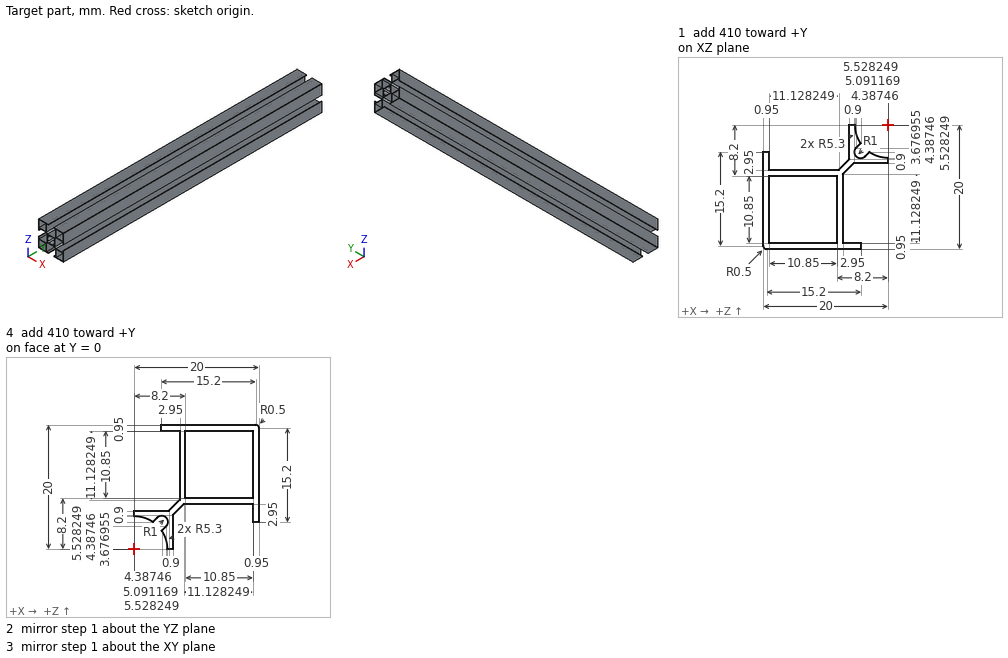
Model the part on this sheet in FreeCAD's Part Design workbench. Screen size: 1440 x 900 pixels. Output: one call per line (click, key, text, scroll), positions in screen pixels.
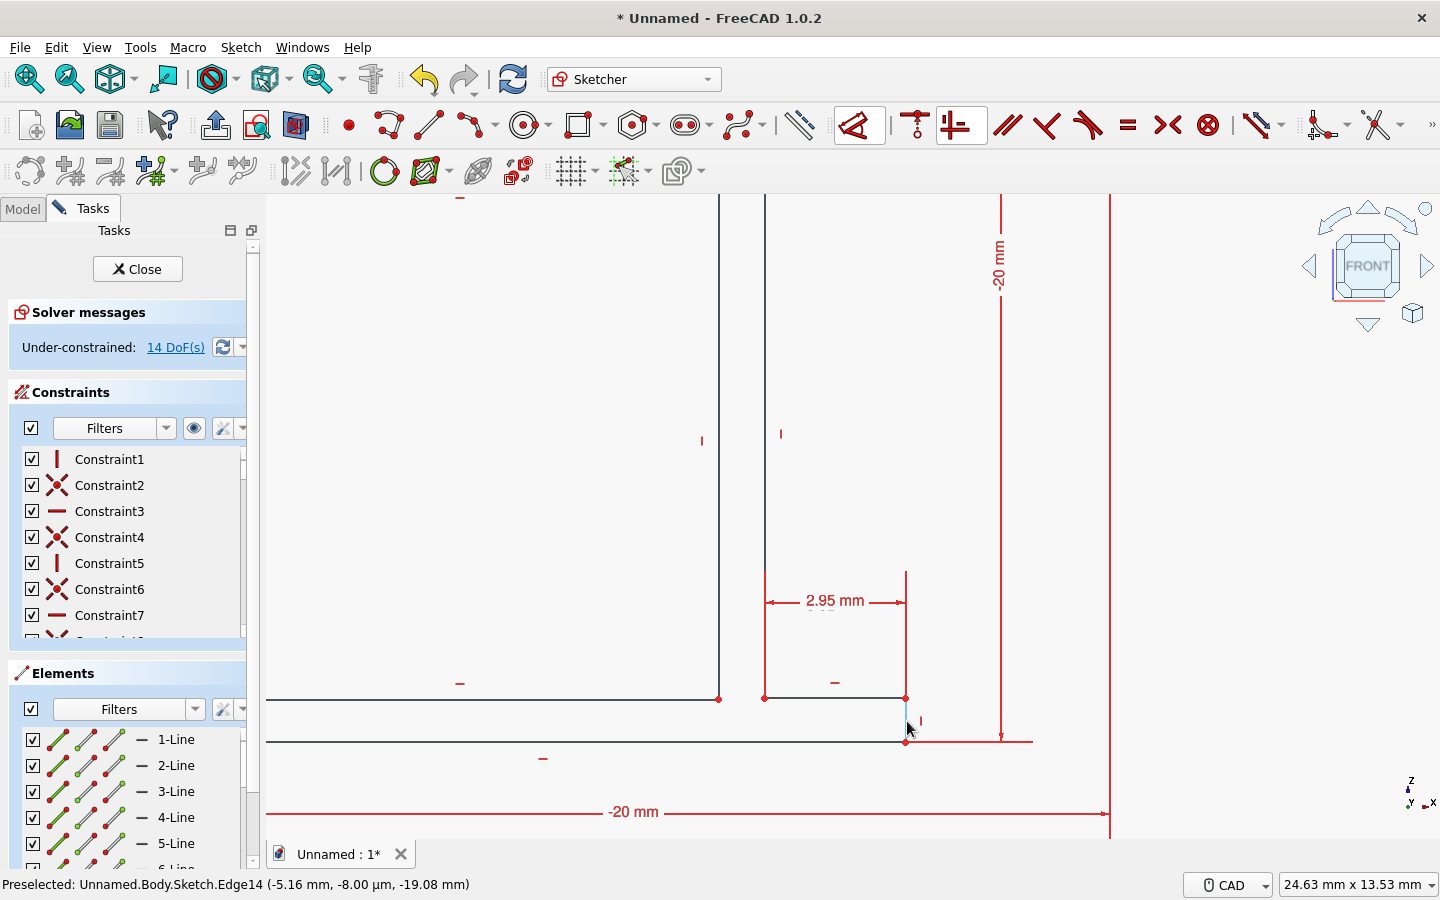
click(906, 720)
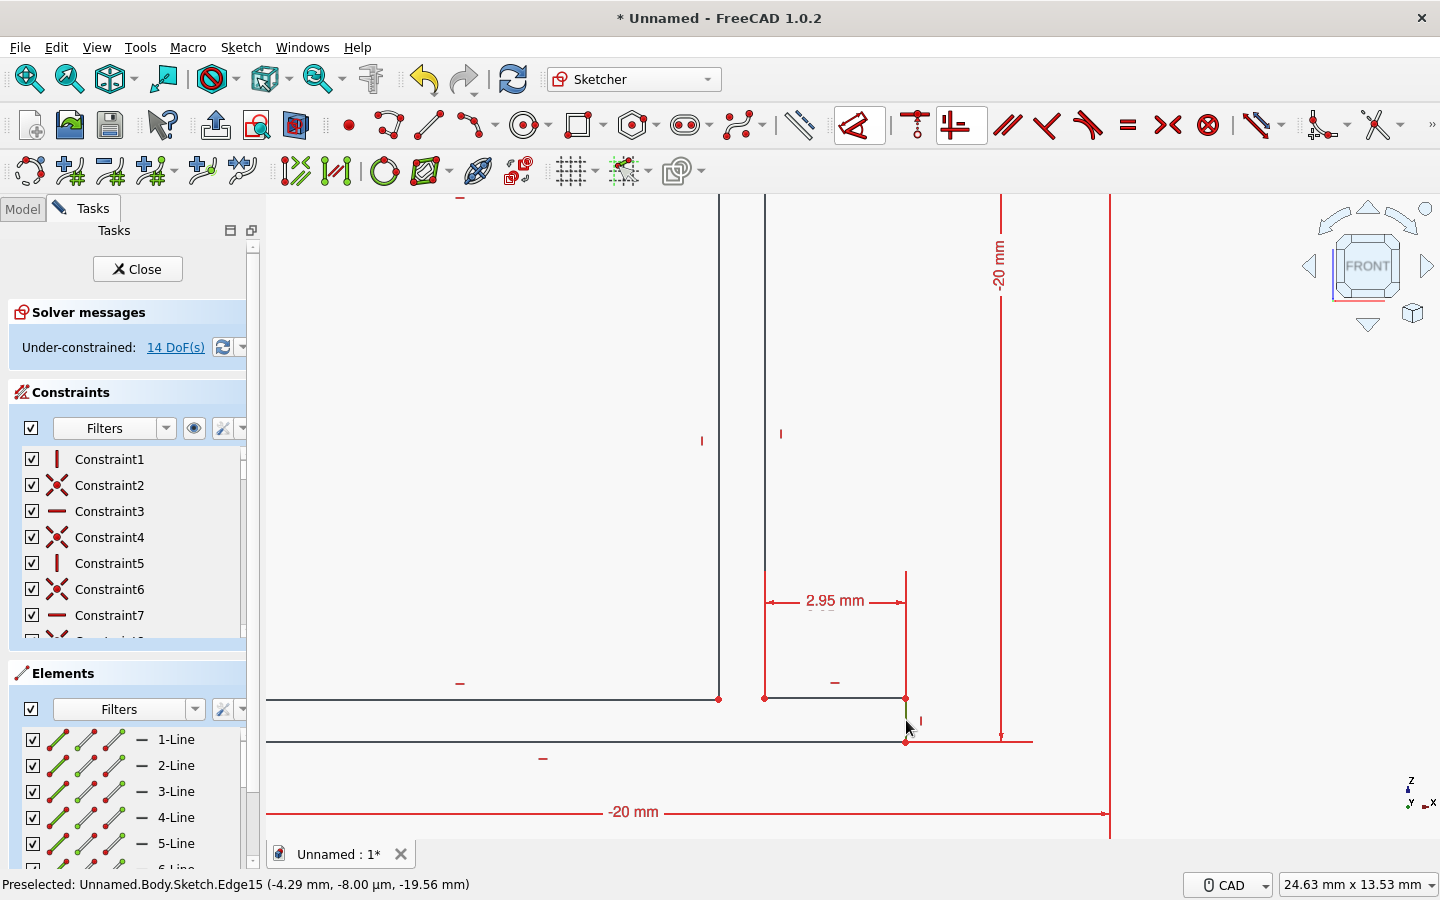
click(880, 126)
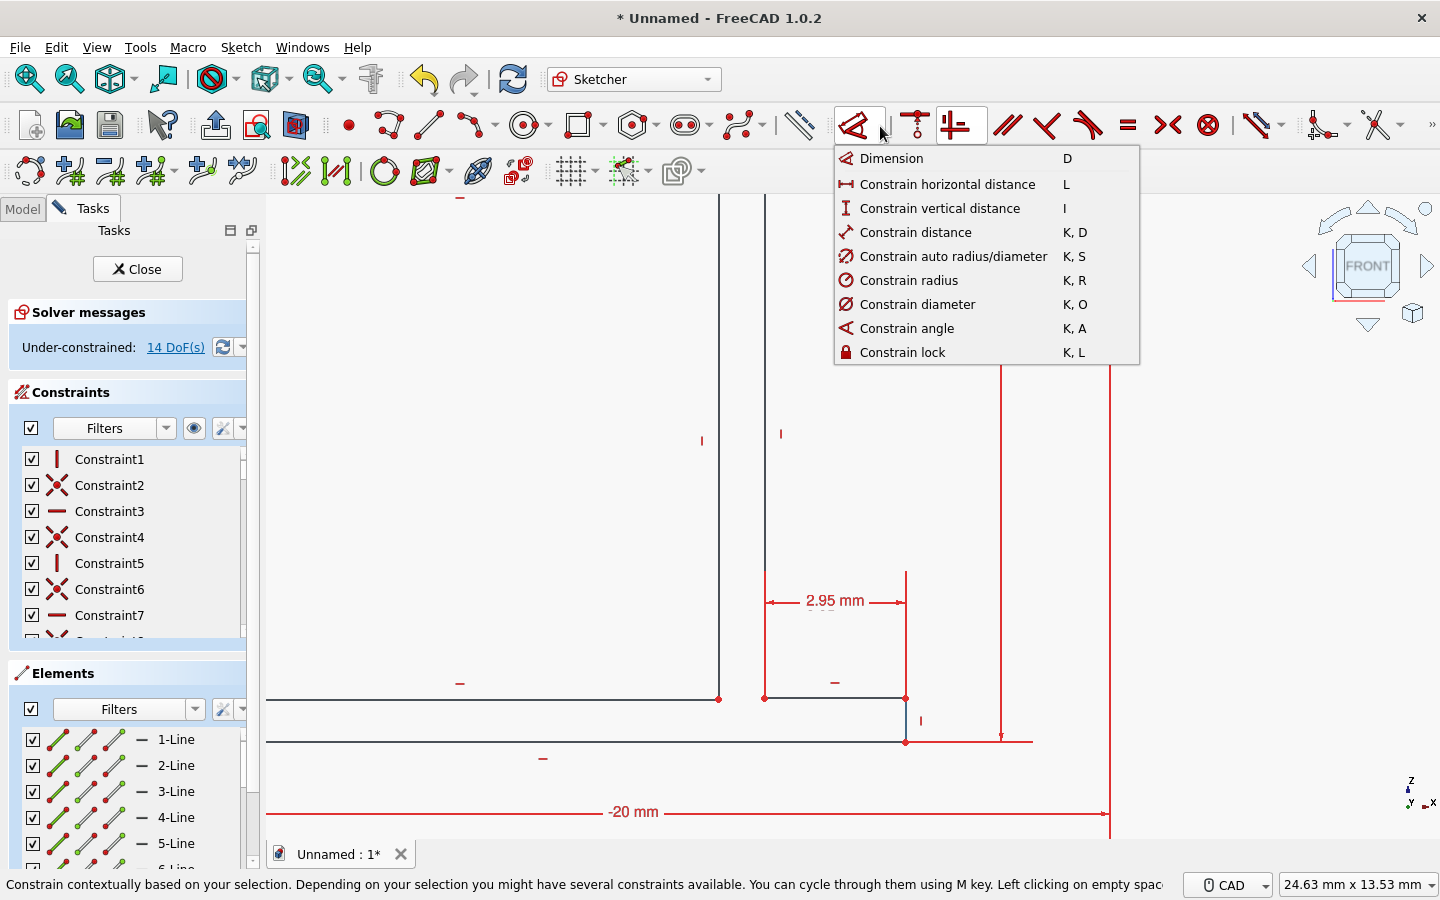
click(987, 208)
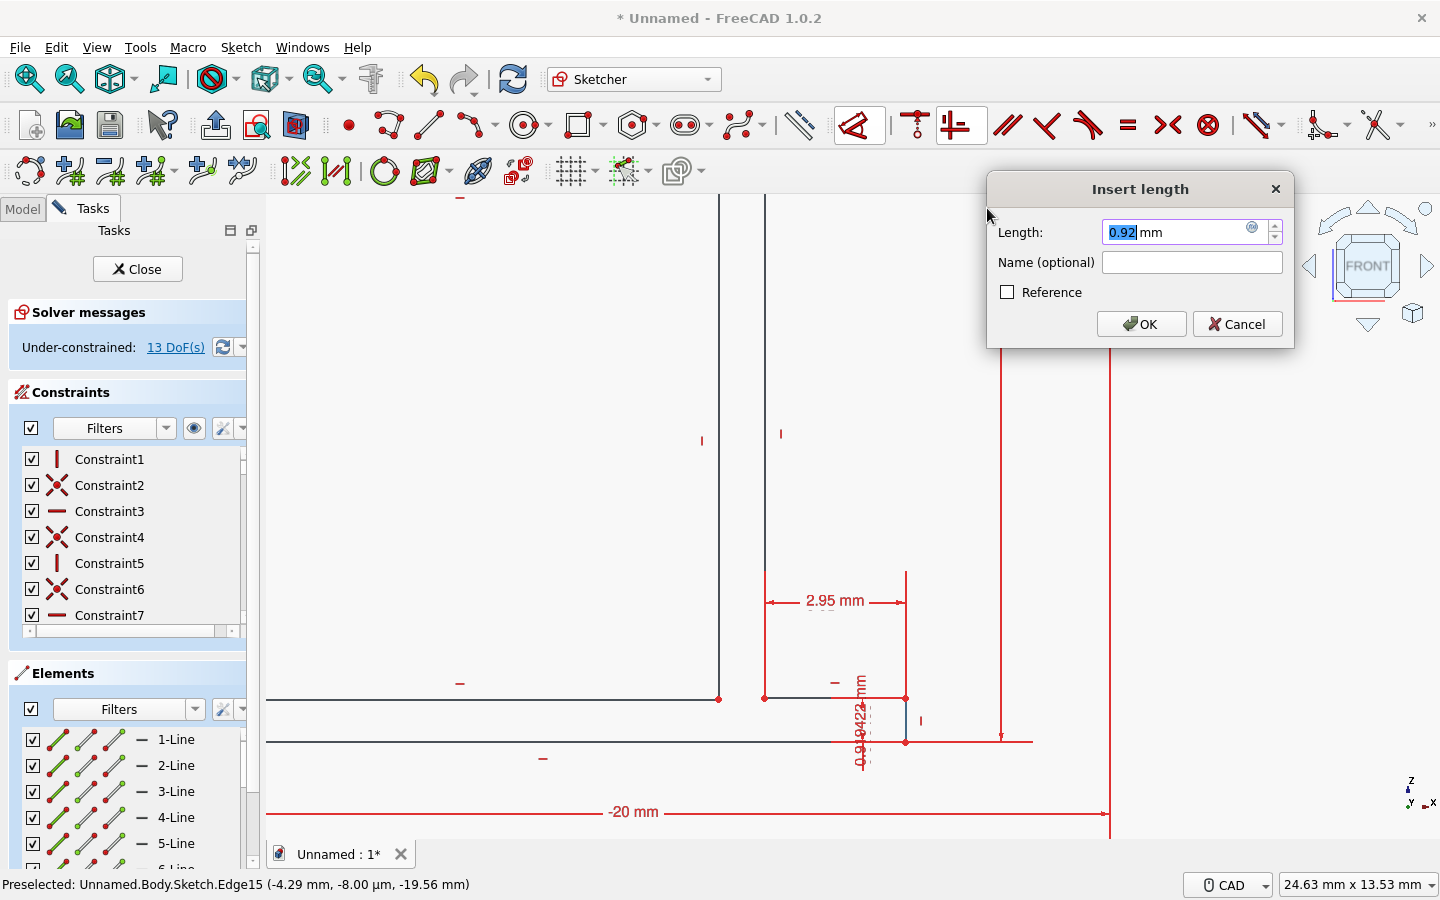
text(0.95)
key(Return)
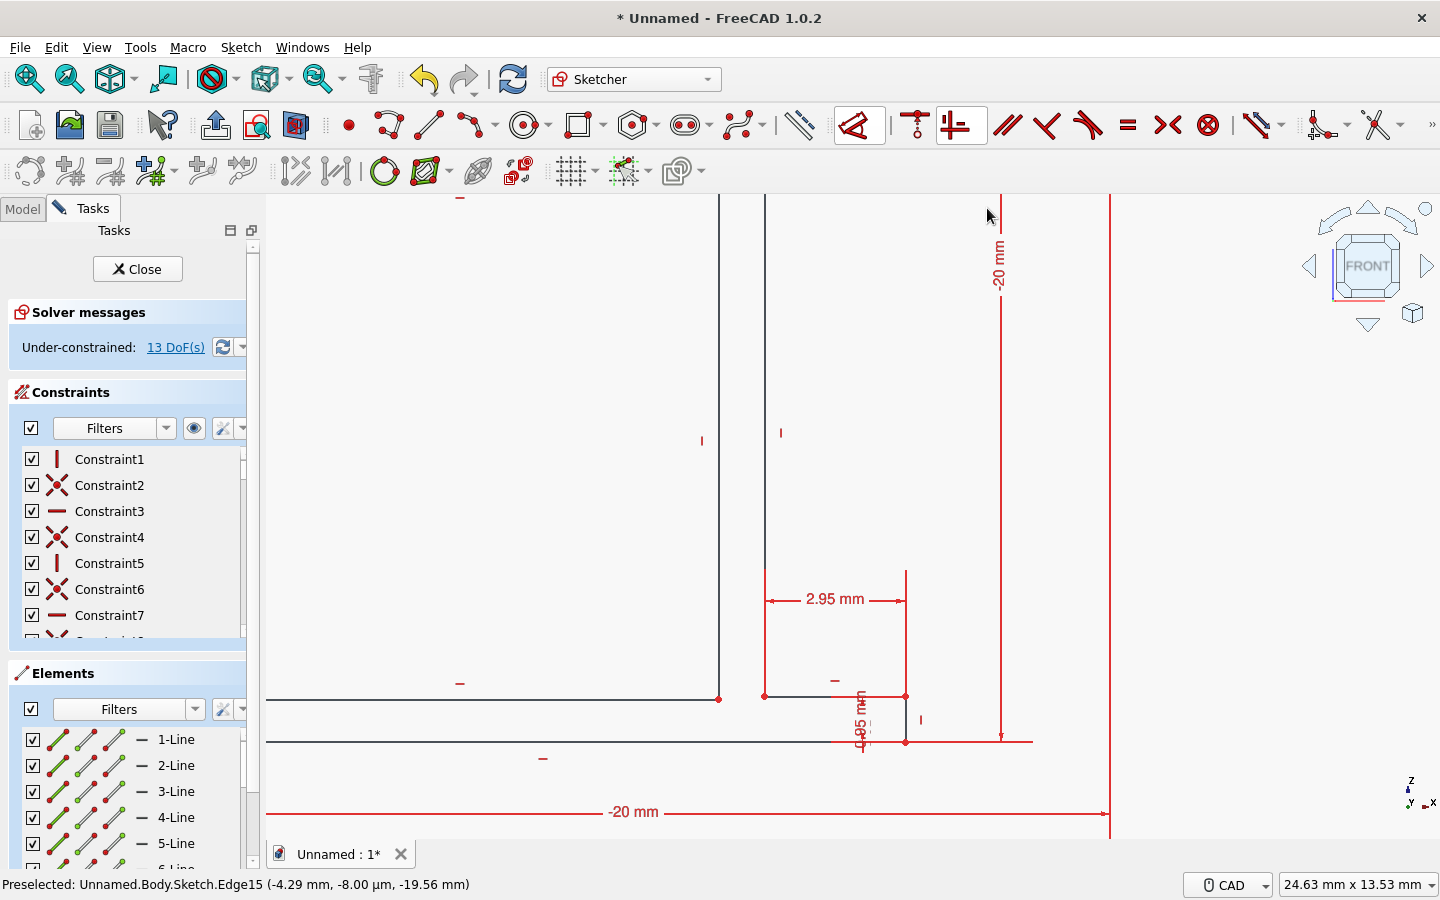
click(688, 742)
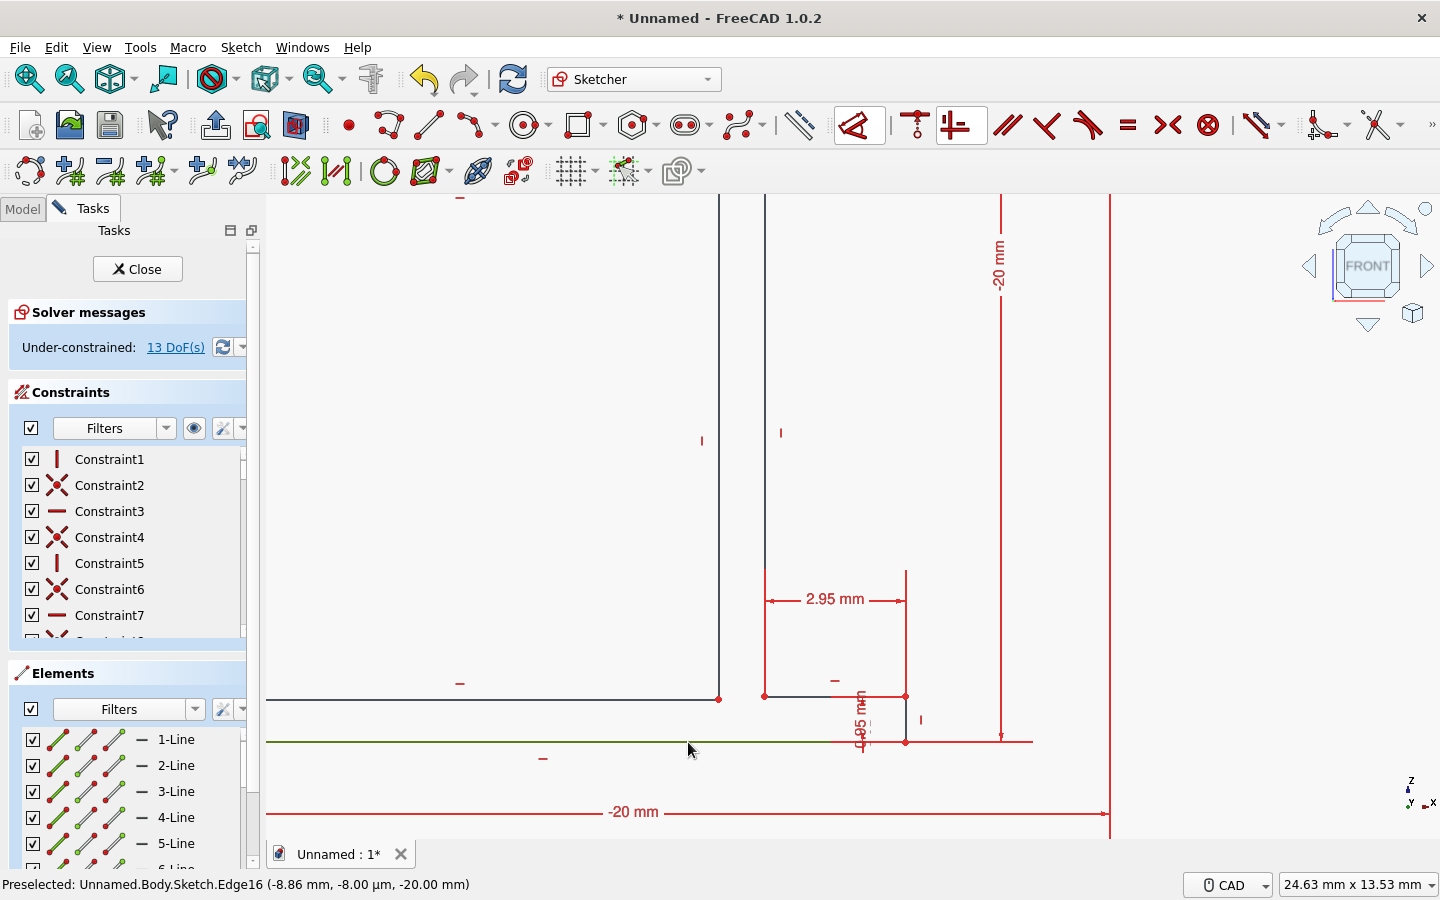
click(880, 126)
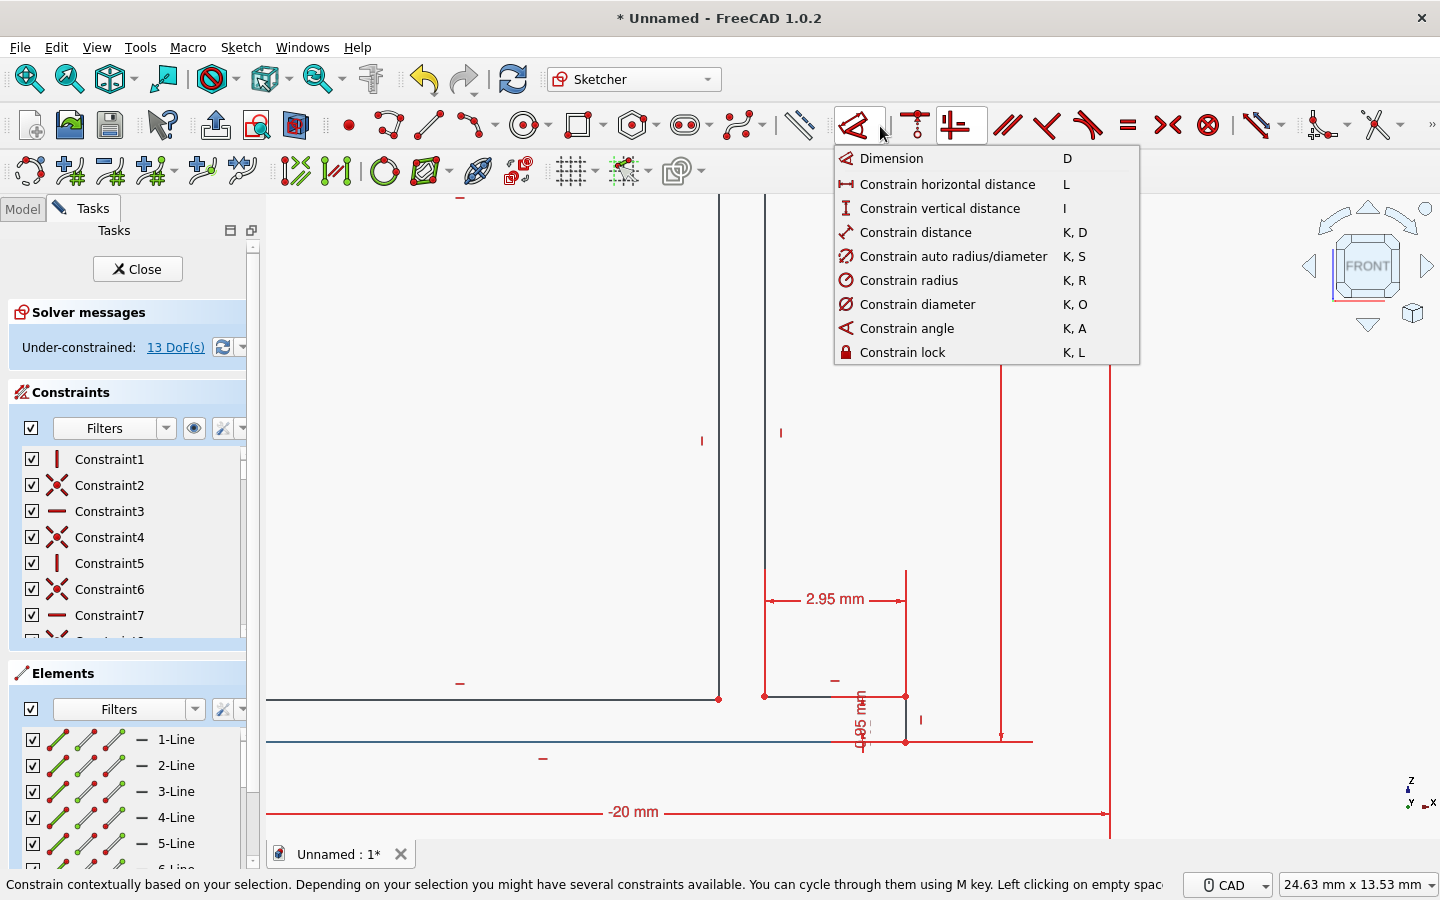
click(987, 184)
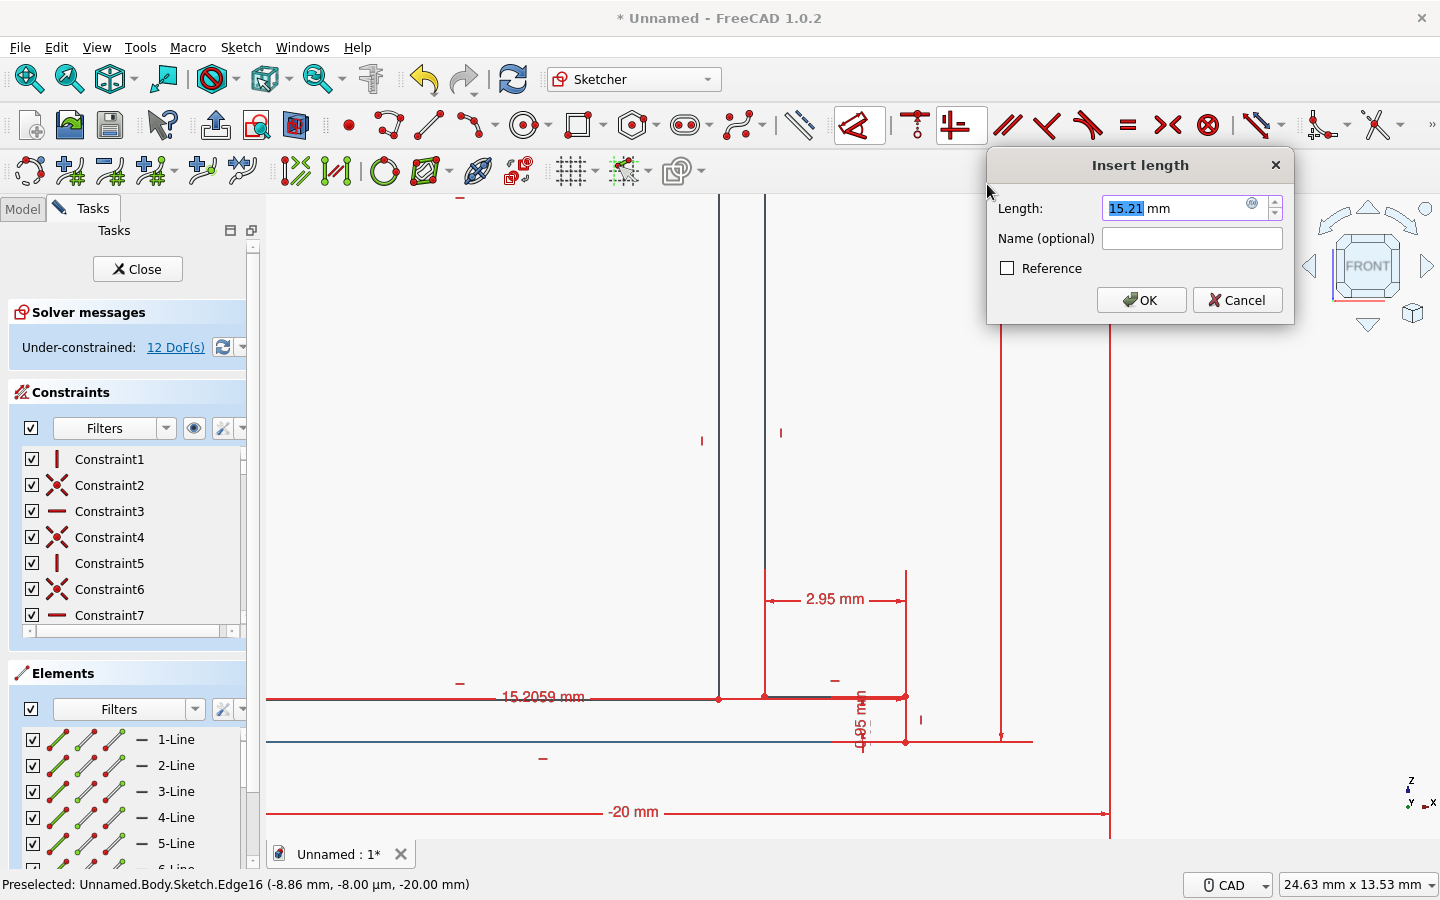
text(15.2)
key(Return)